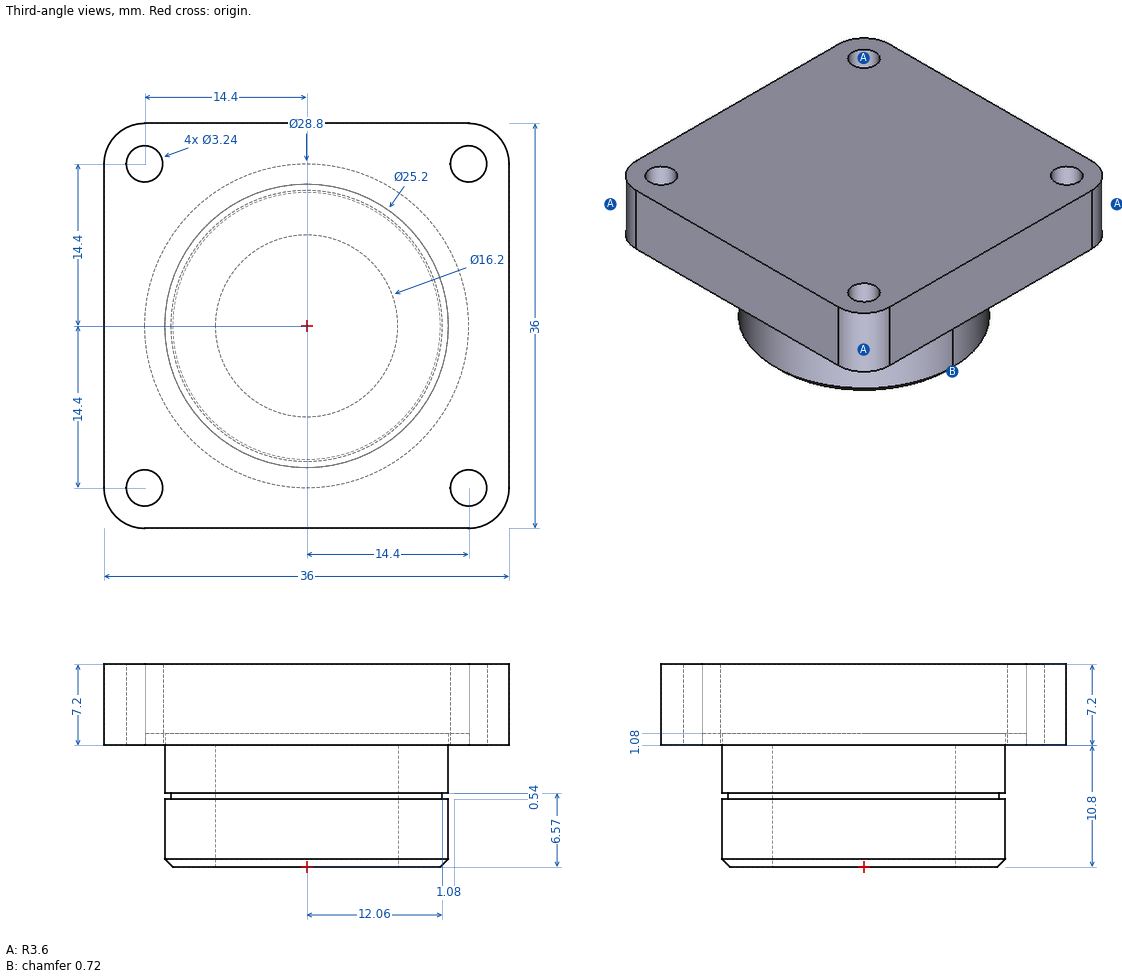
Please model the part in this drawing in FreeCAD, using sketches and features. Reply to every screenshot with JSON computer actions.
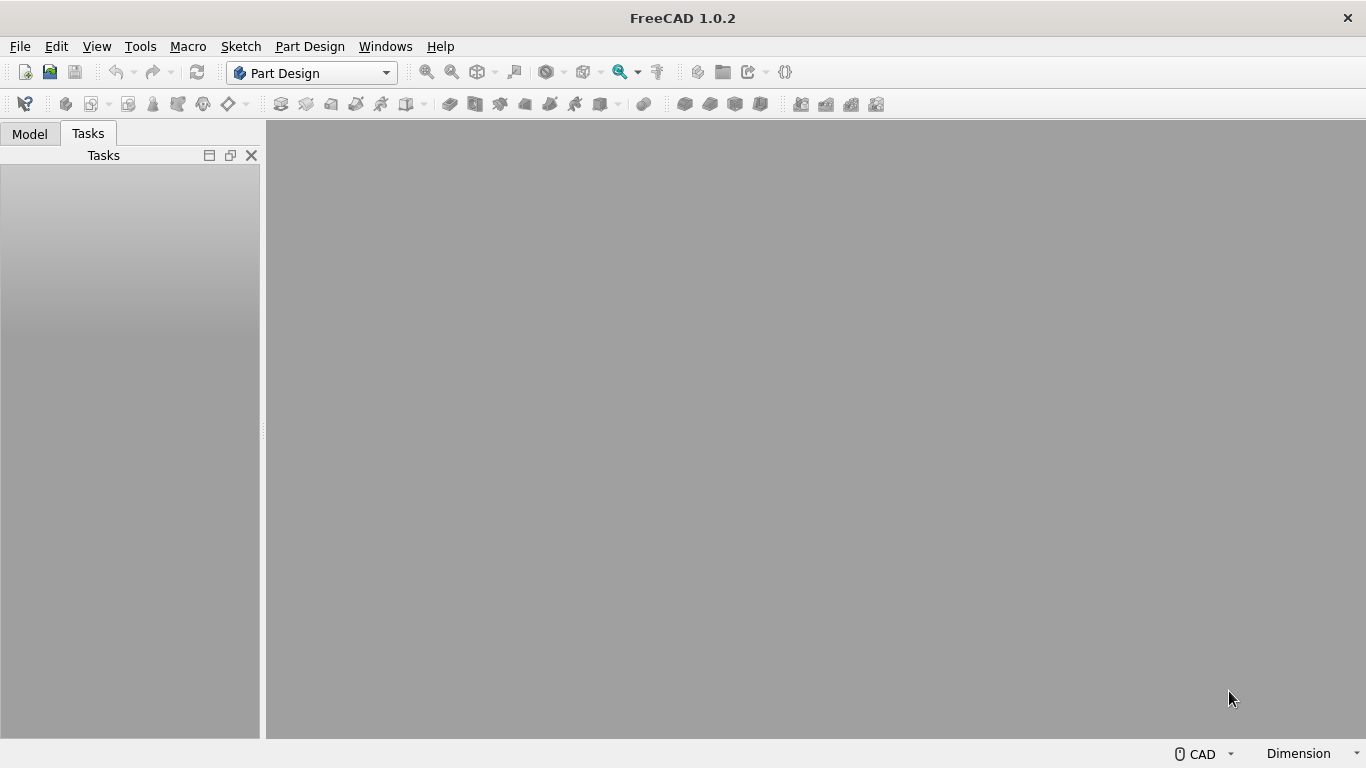
{"action": "key", "text": "ctrl+n"}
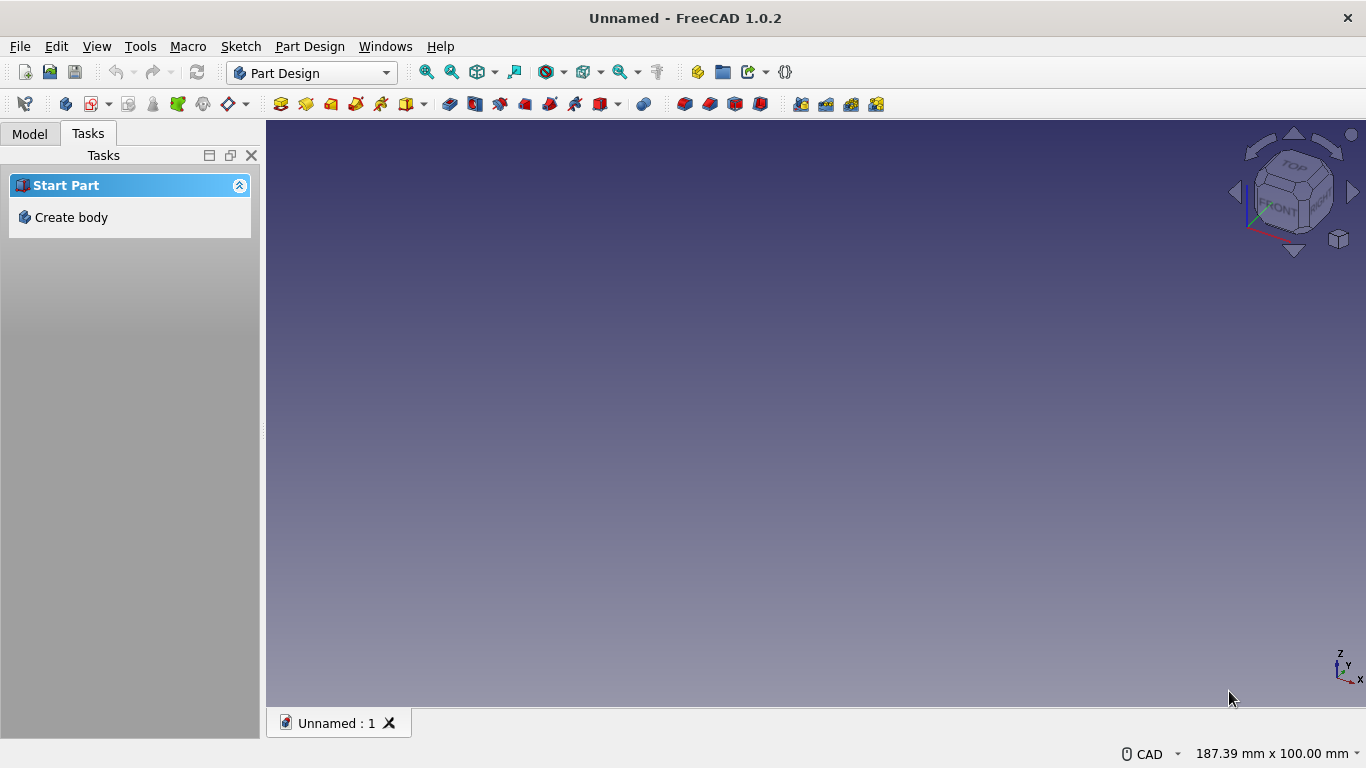
{"action": "left_click", "coordinate": [90, 104]}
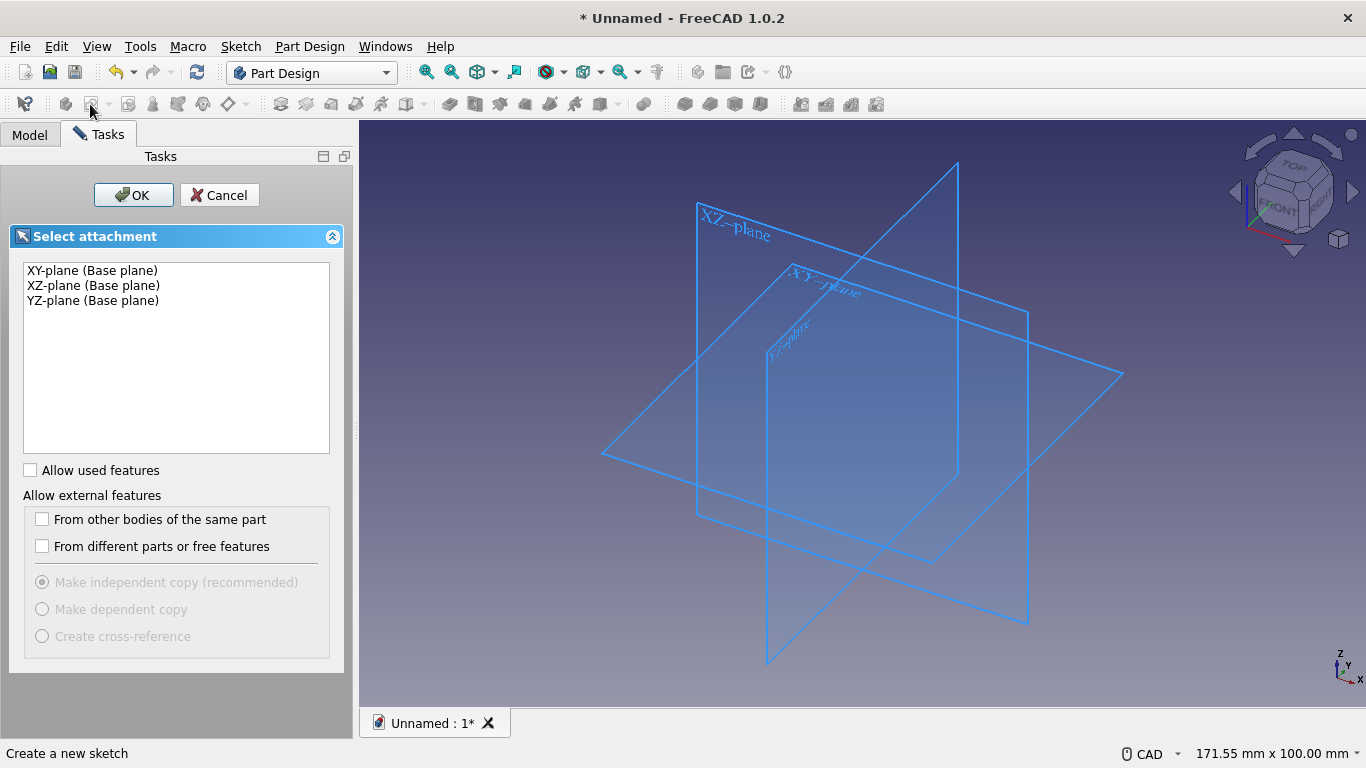
{"action": "left_click", "coordinate": [84, 270]}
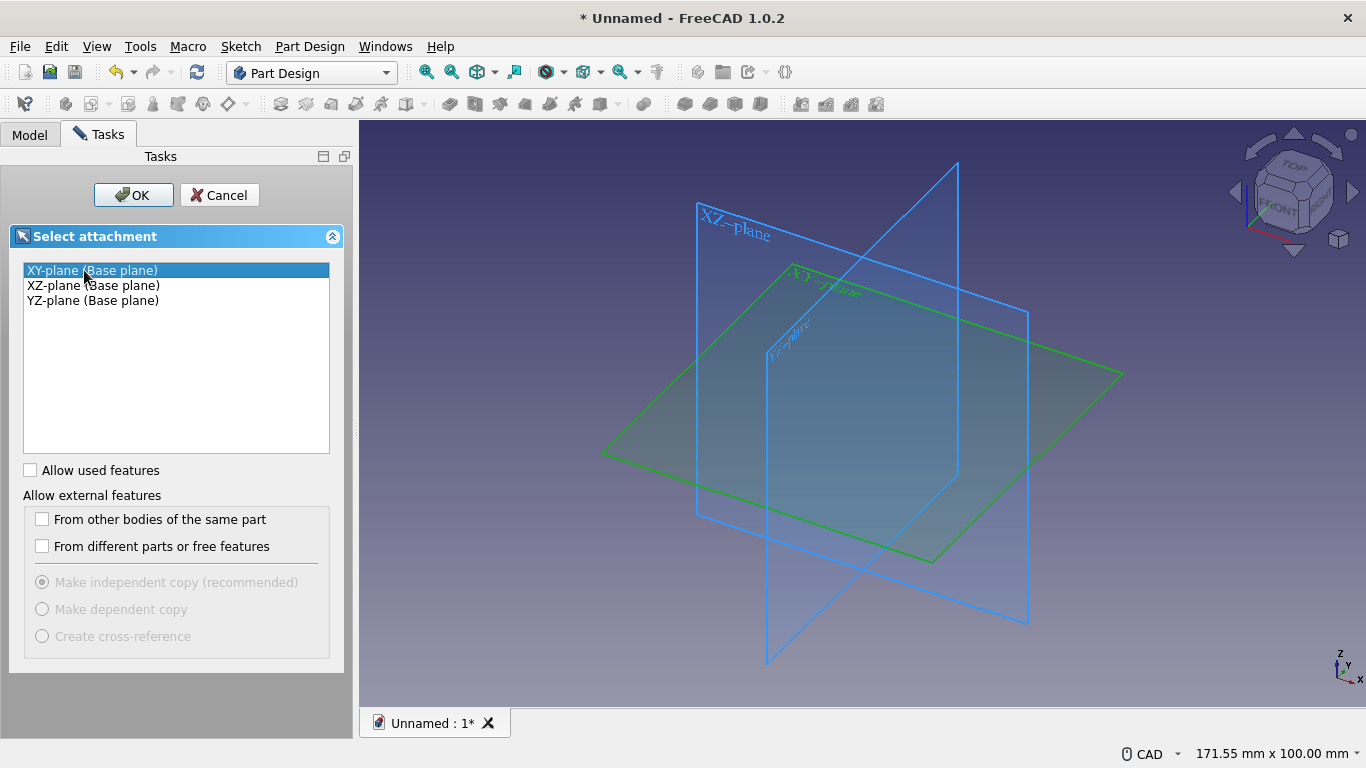
{"action": "left_click", "coordinate": [134, 195]}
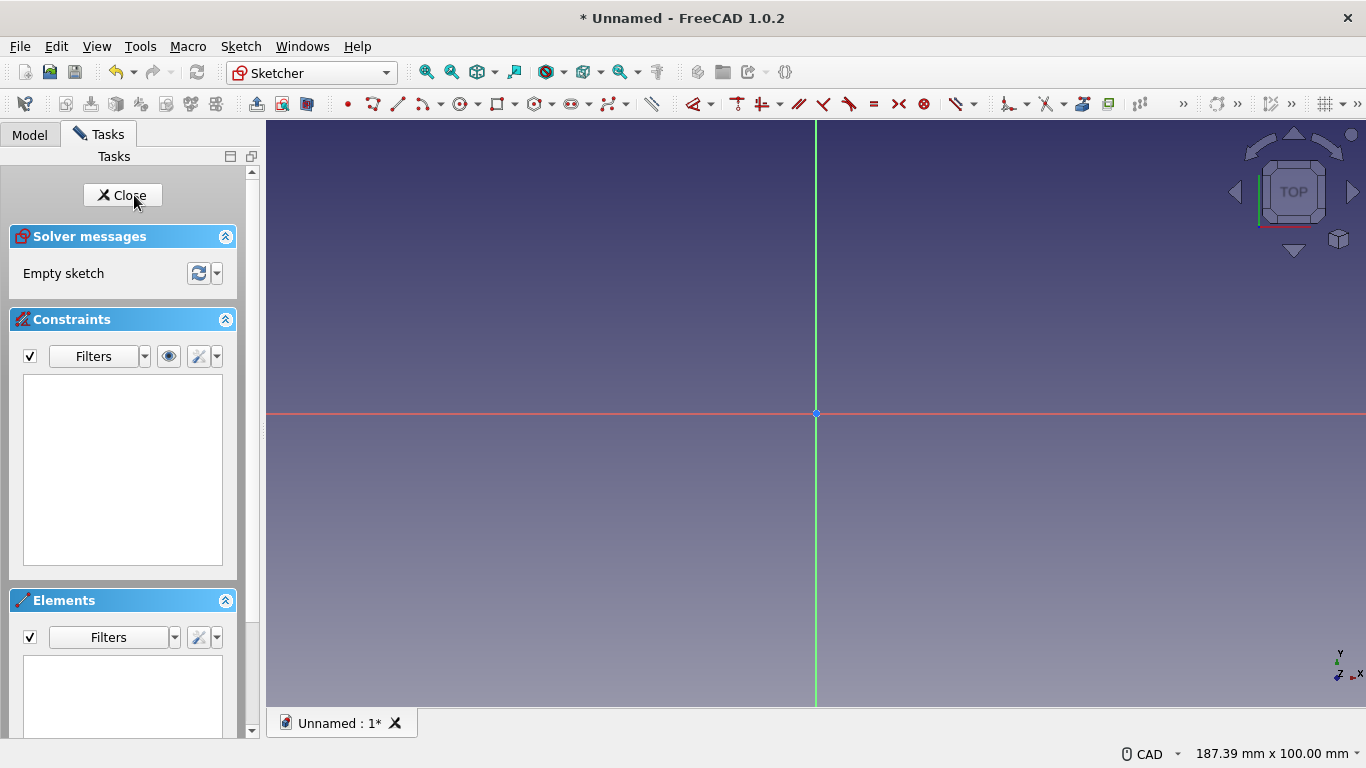
{"action": "scroll", "coordinate": [856, 414], "scroll_direction": "up", "scroll_amount": 5}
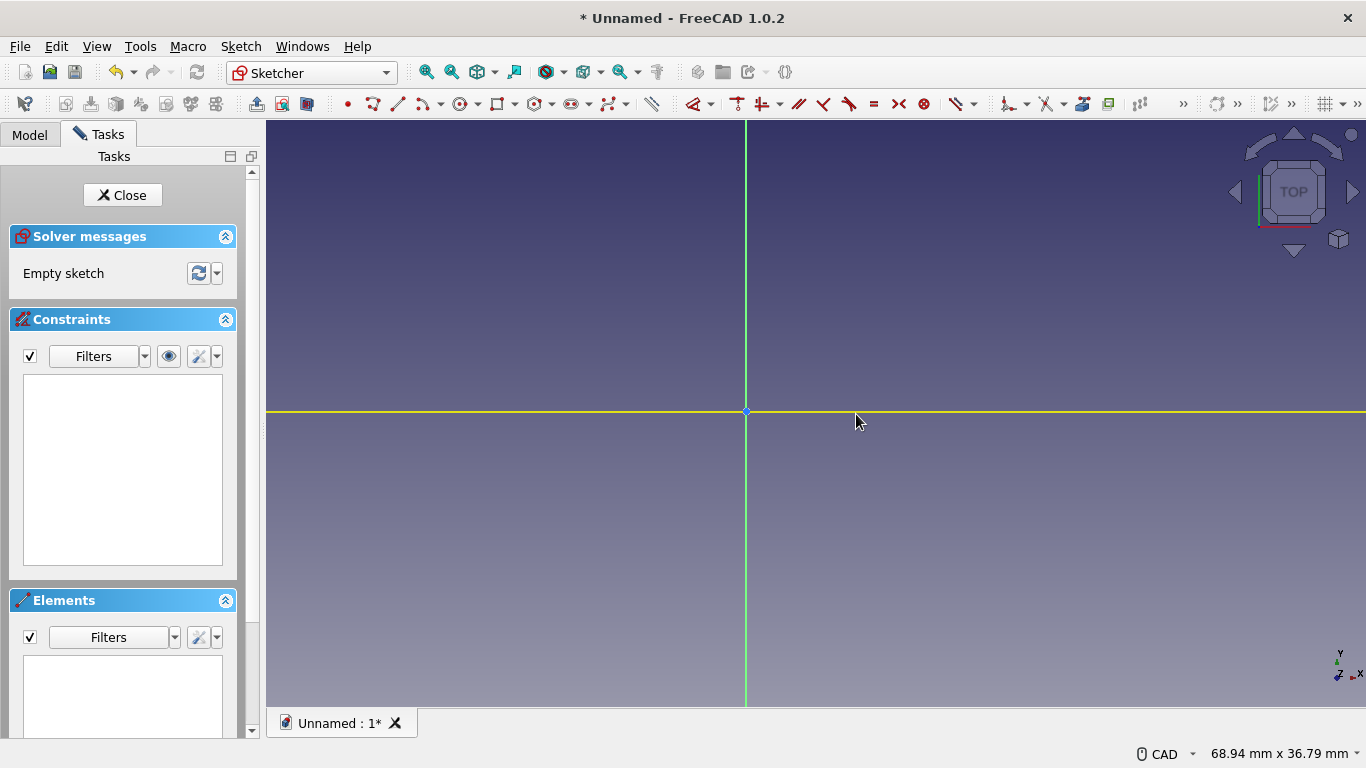
{"action": "key", "text": "g c"}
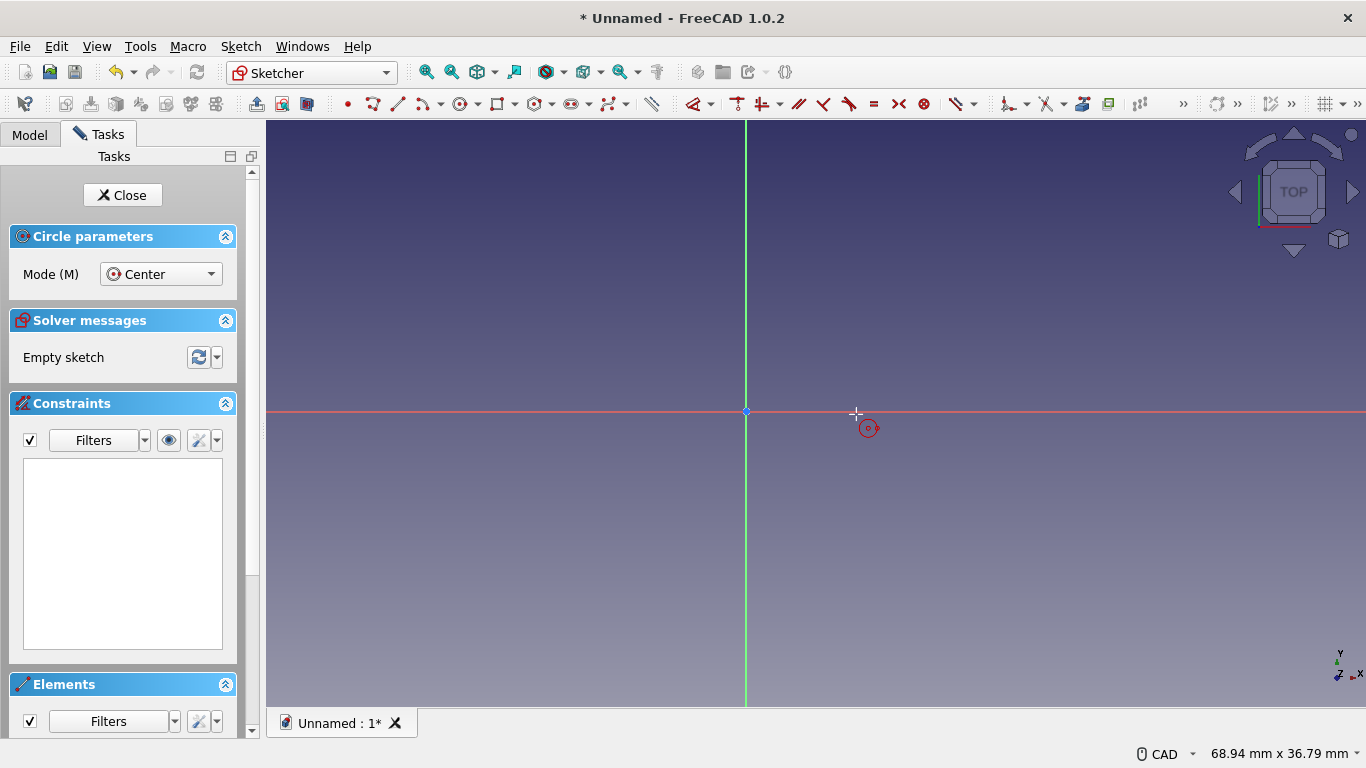
{"action": "left_click", "coordinate": [746, 412]}
{"action": "mouse_move", "coordinate": [889, 270]}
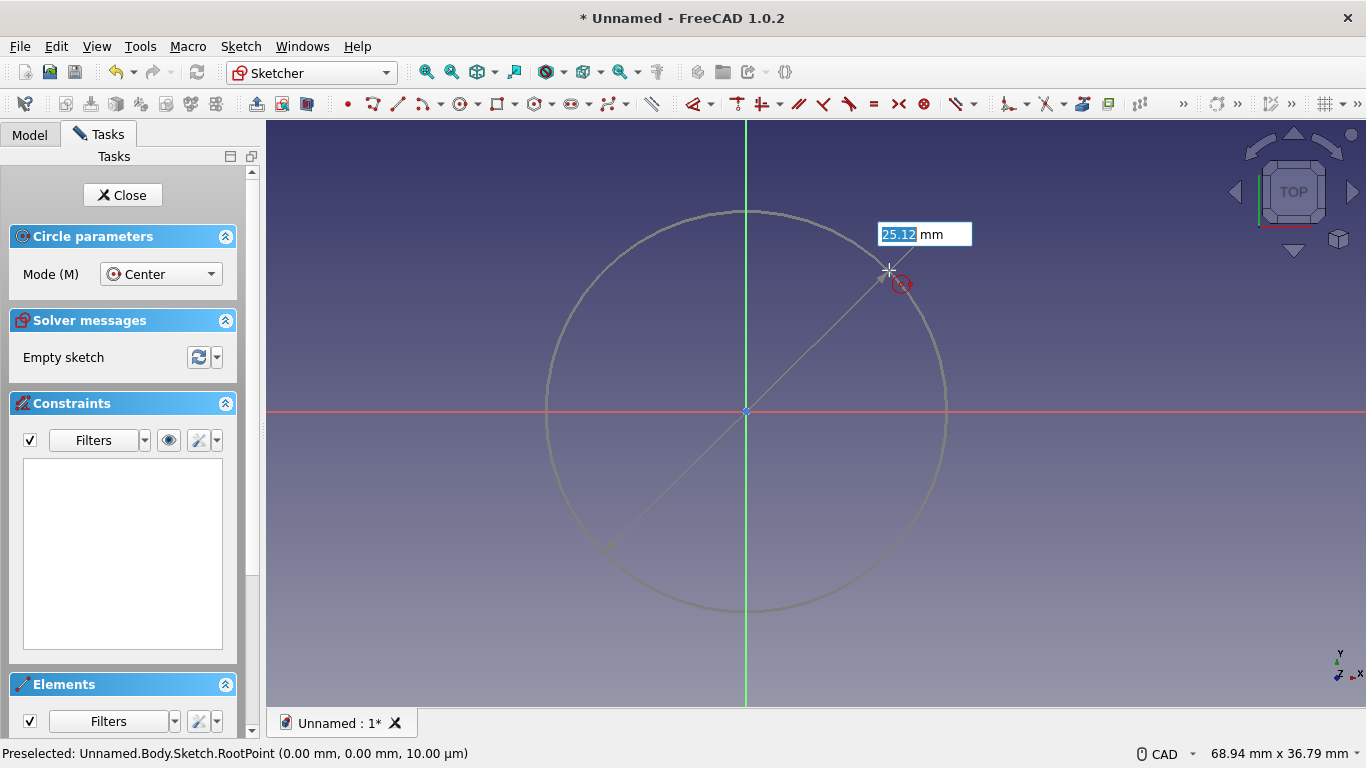
{"action": "type", "text": "25.2"}
{"action": "key", "text": "Return"}
{"action": "key", "text": "Escape"}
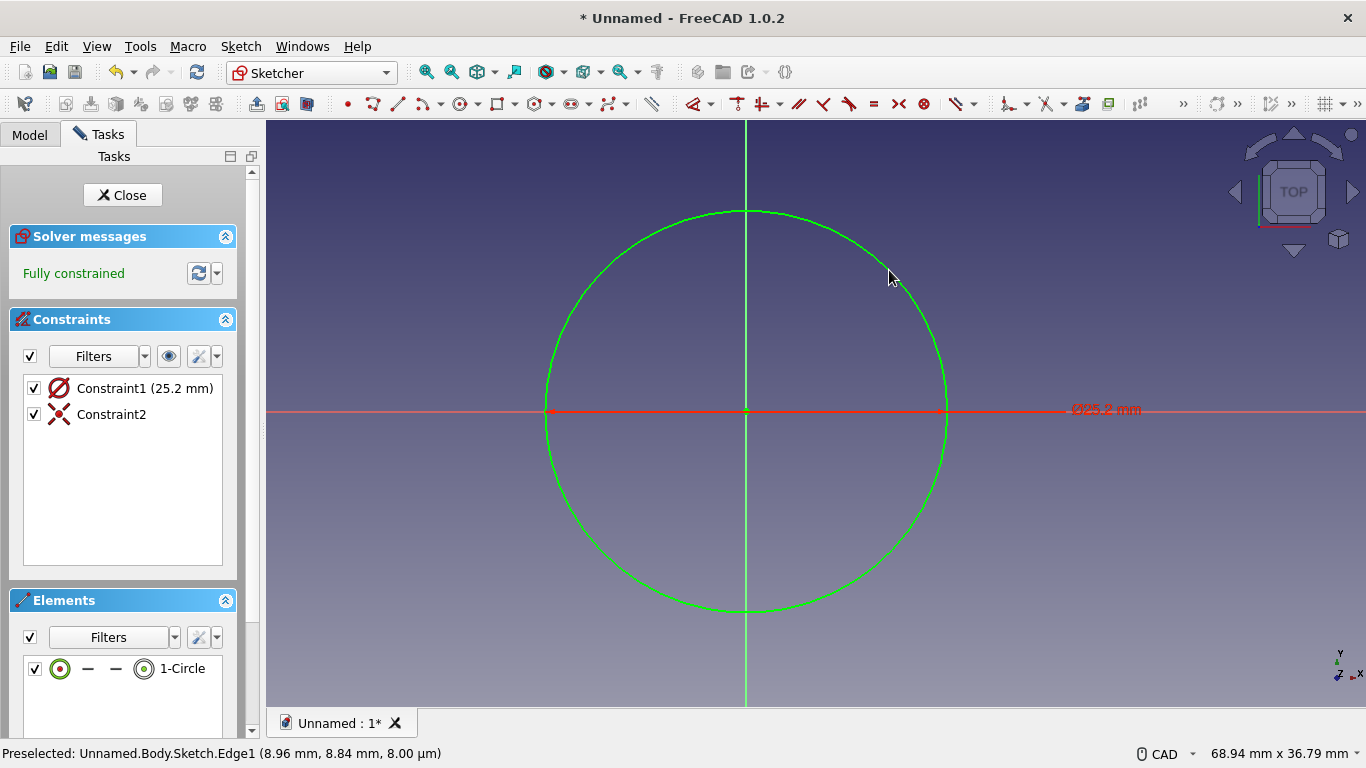
{"action": "left_click", "coordinate": [123, 195]}